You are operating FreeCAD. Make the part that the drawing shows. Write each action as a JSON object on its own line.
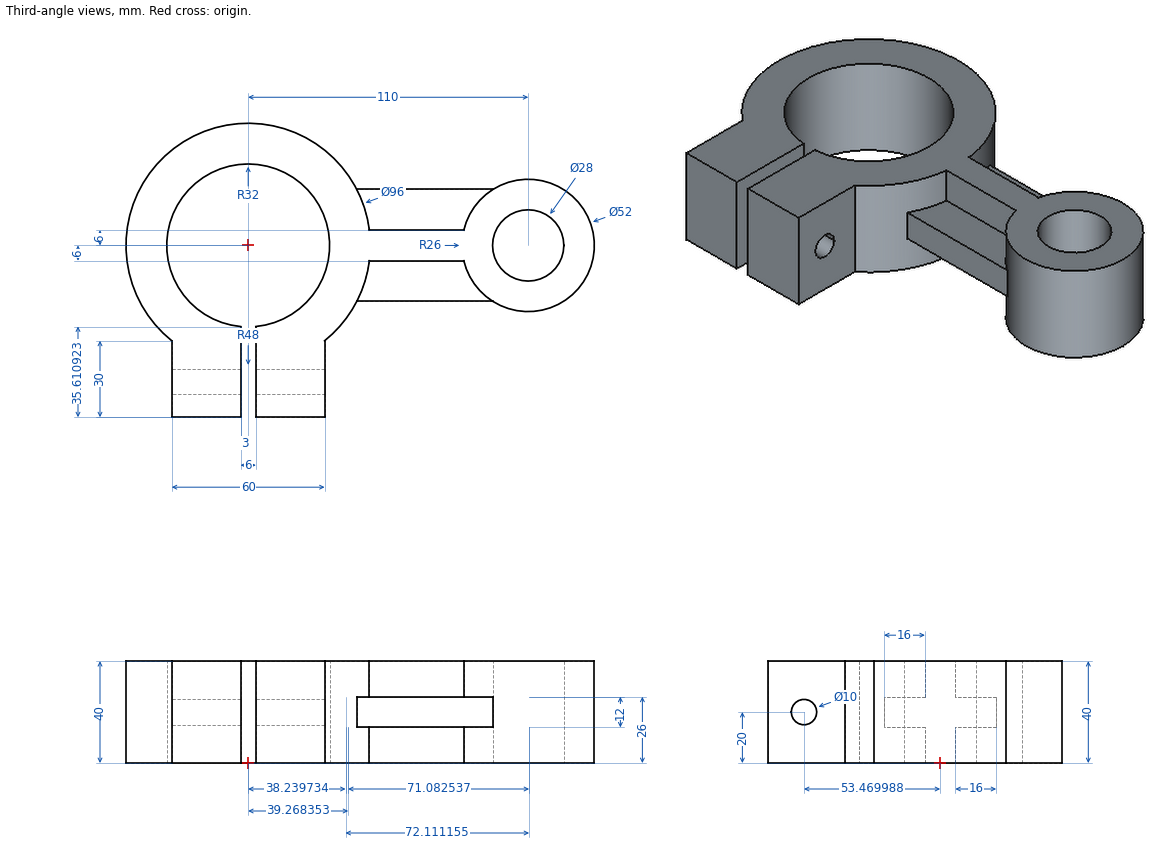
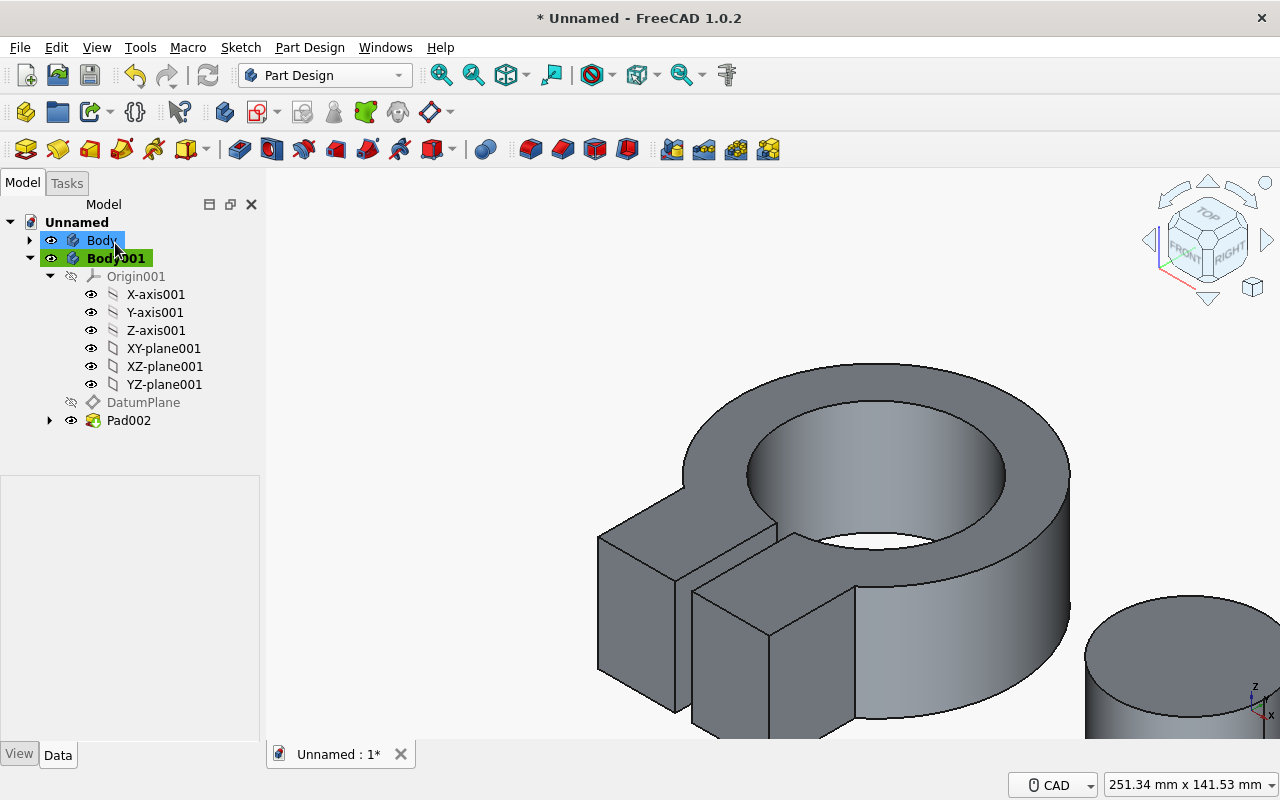
{"action": "left_click", "coordinate": [442, 76]}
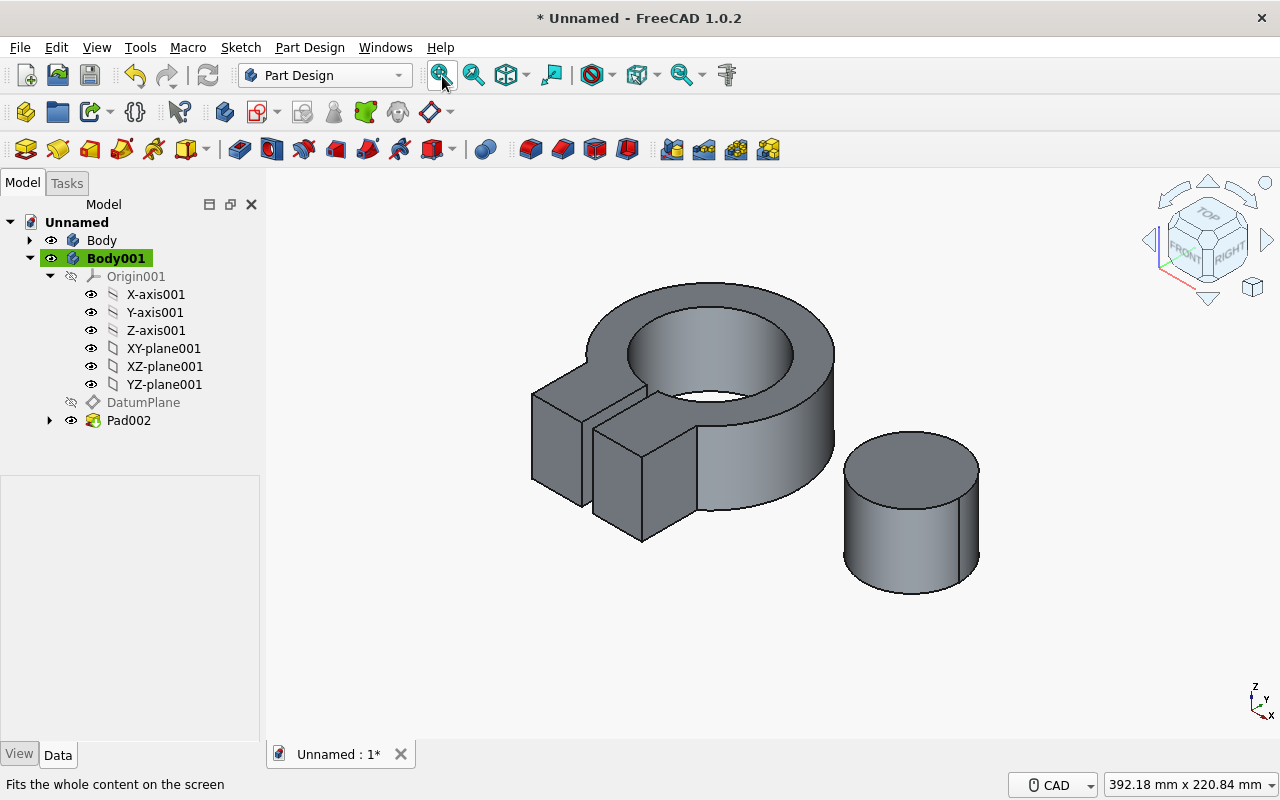
{"action": "double_click", "coordinate": [96, 240]}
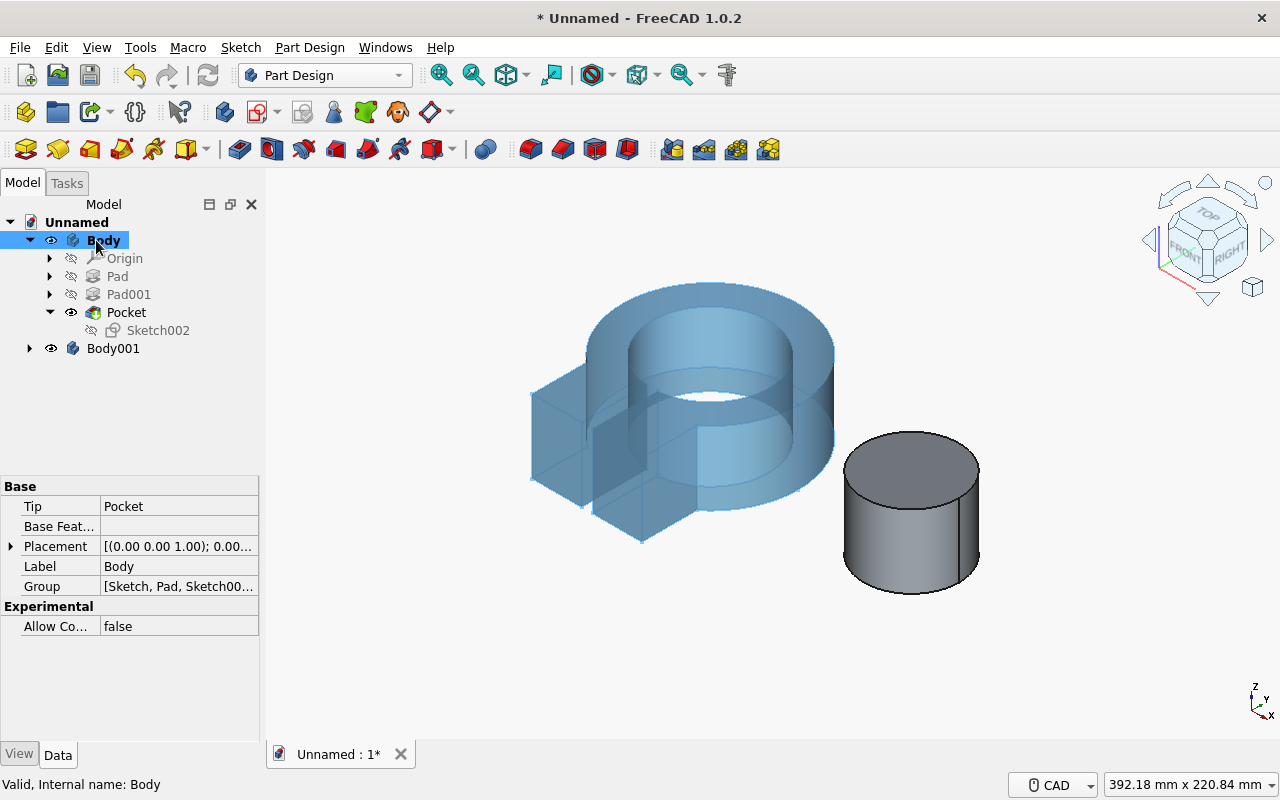
{"action": "left_click", "coordinate": [96, 240]}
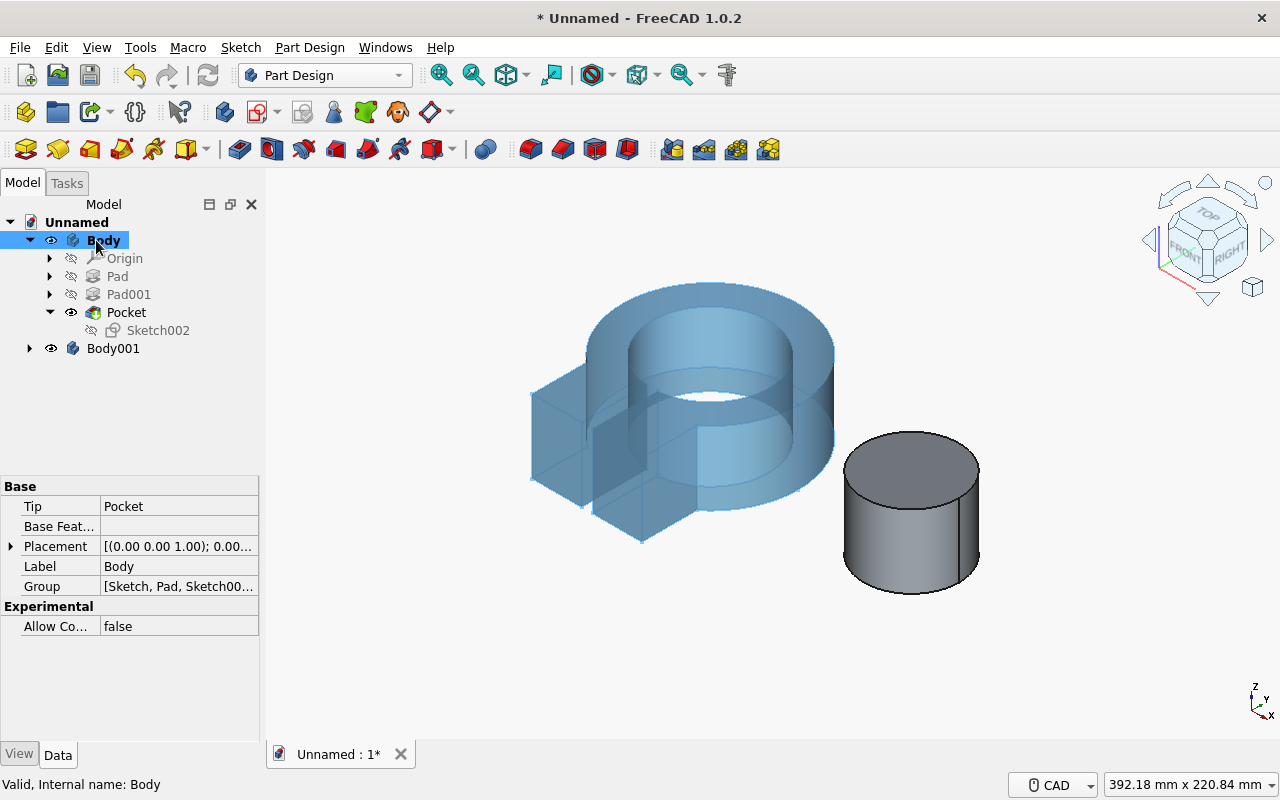
{"action": "left_click", "coordinate": [146, 626]}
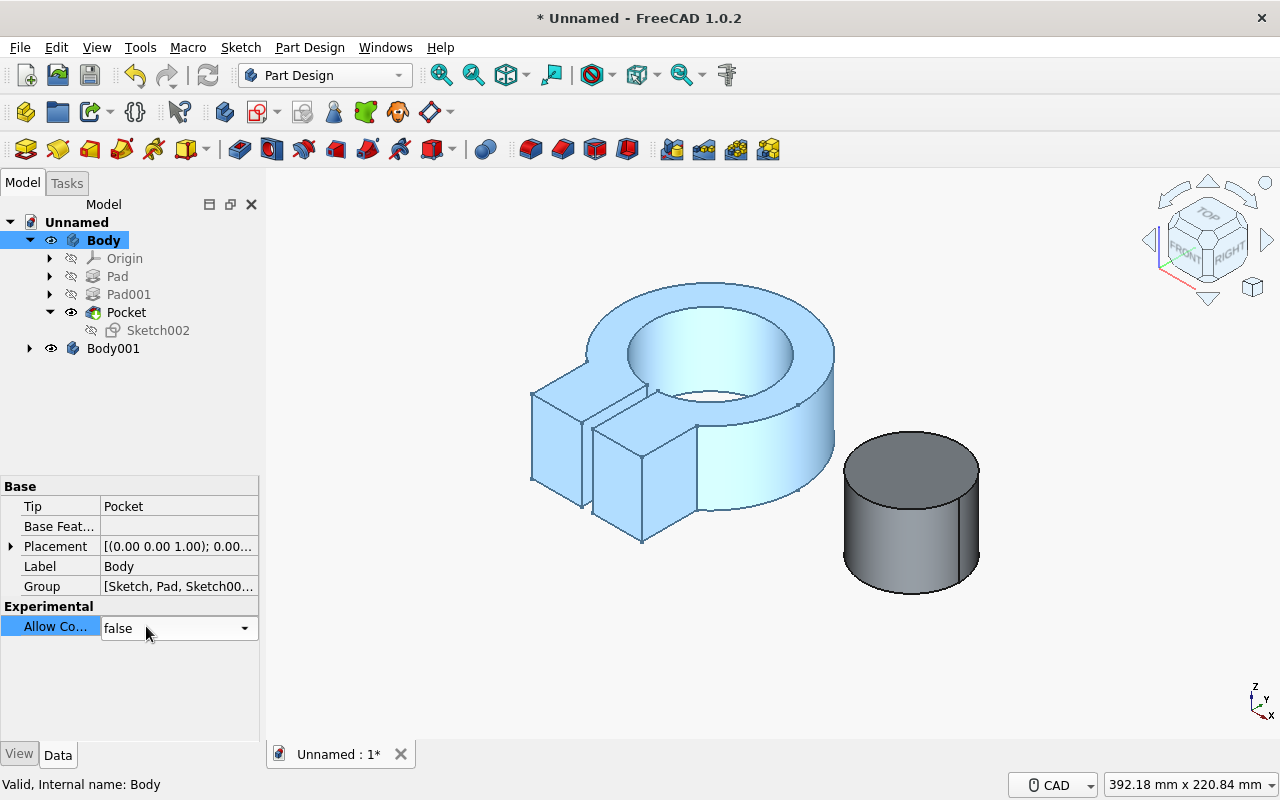
{"action": "left_click", "coordinate": [146, 626]}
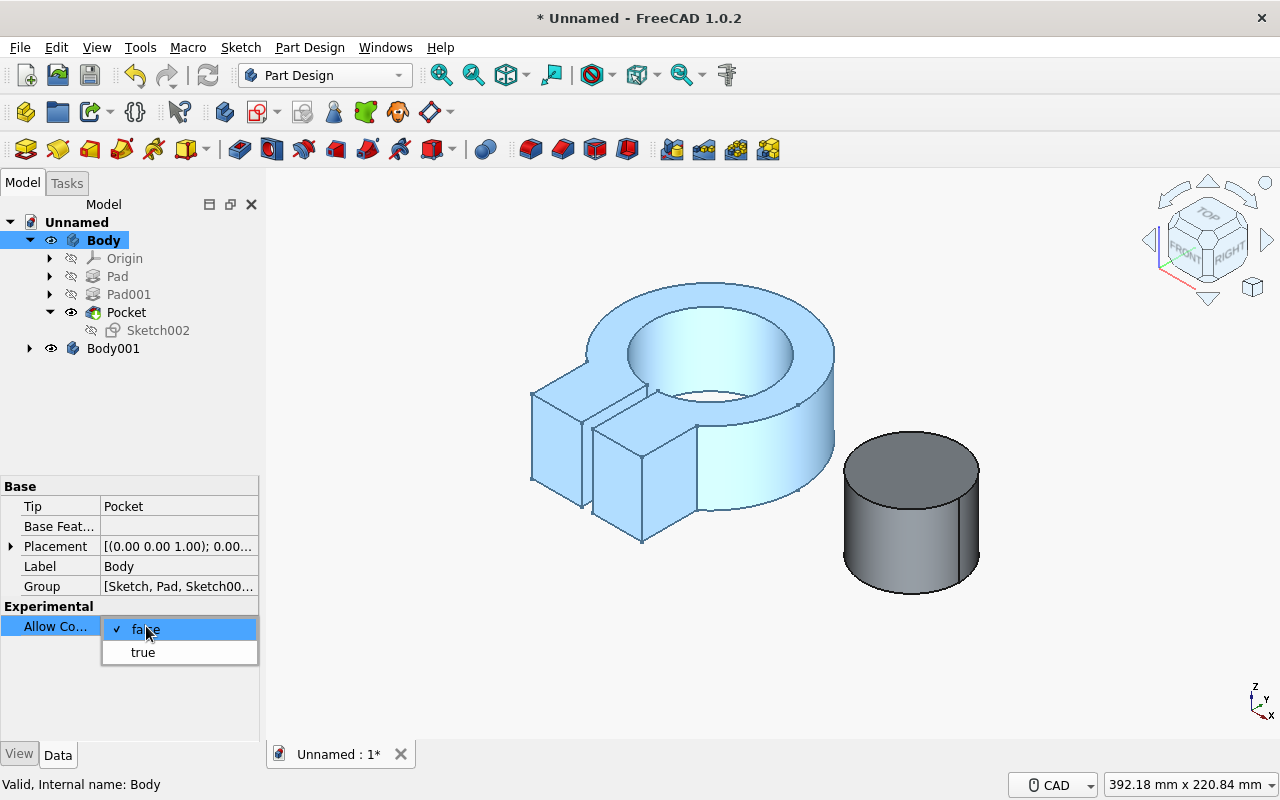
{"action": "left_click", "coordinate": [179, 652]}
{"action": "key", "text": "Return"}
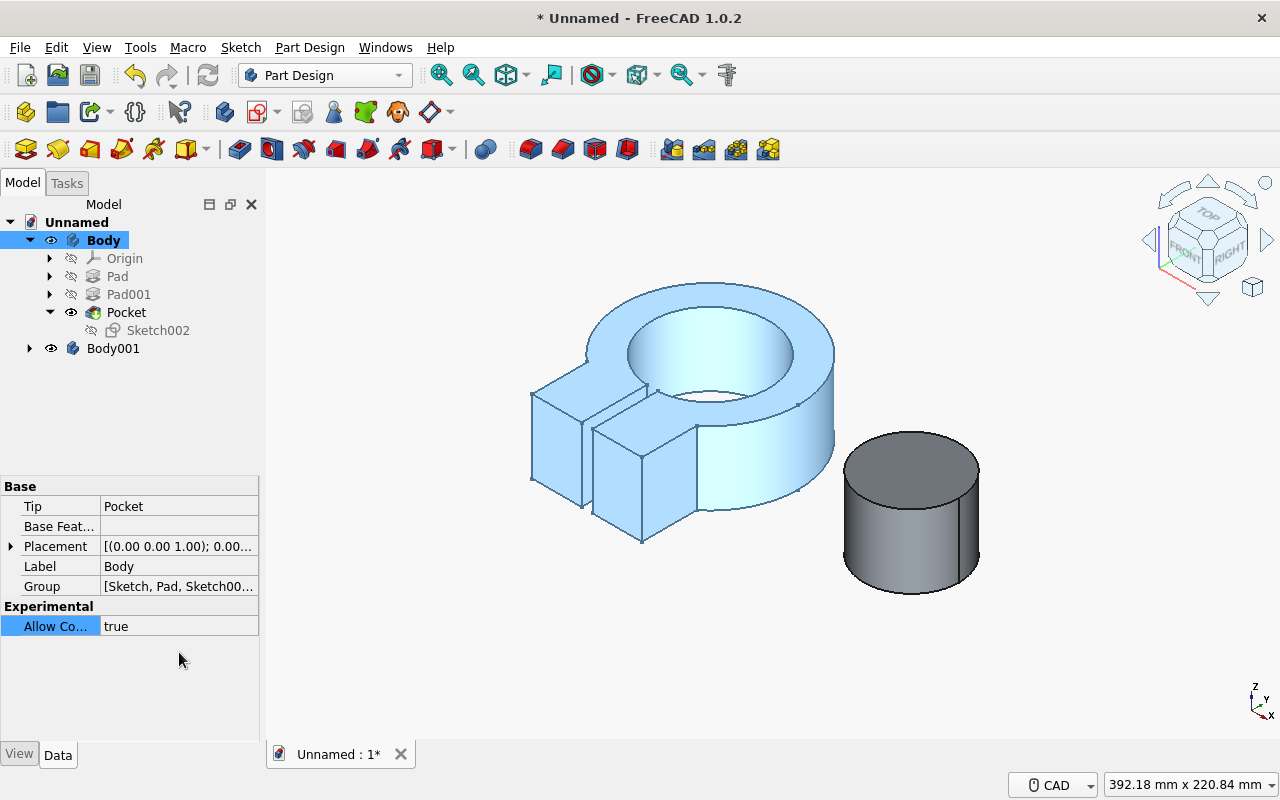
{"action": "left_click", "coordinate": [96, 348]}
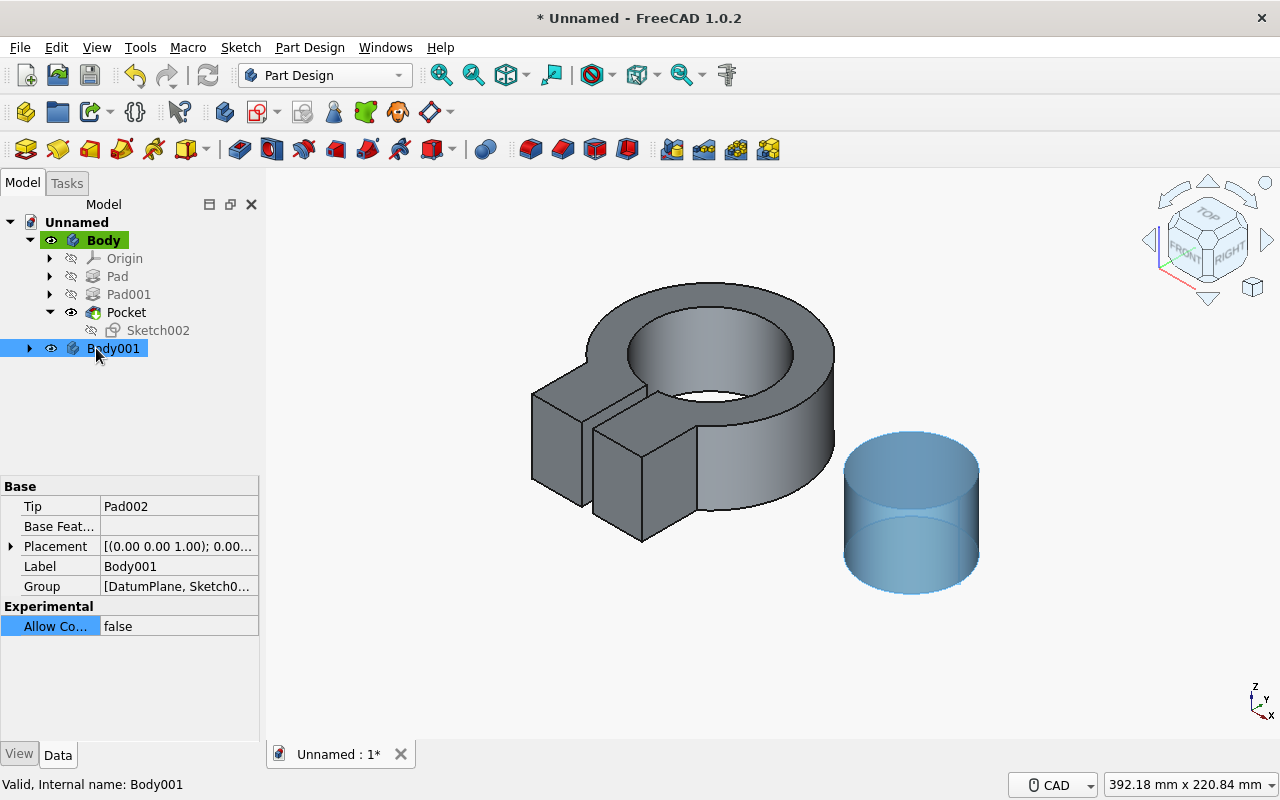
{"action": "left_click", "coordinate": [486, 150]}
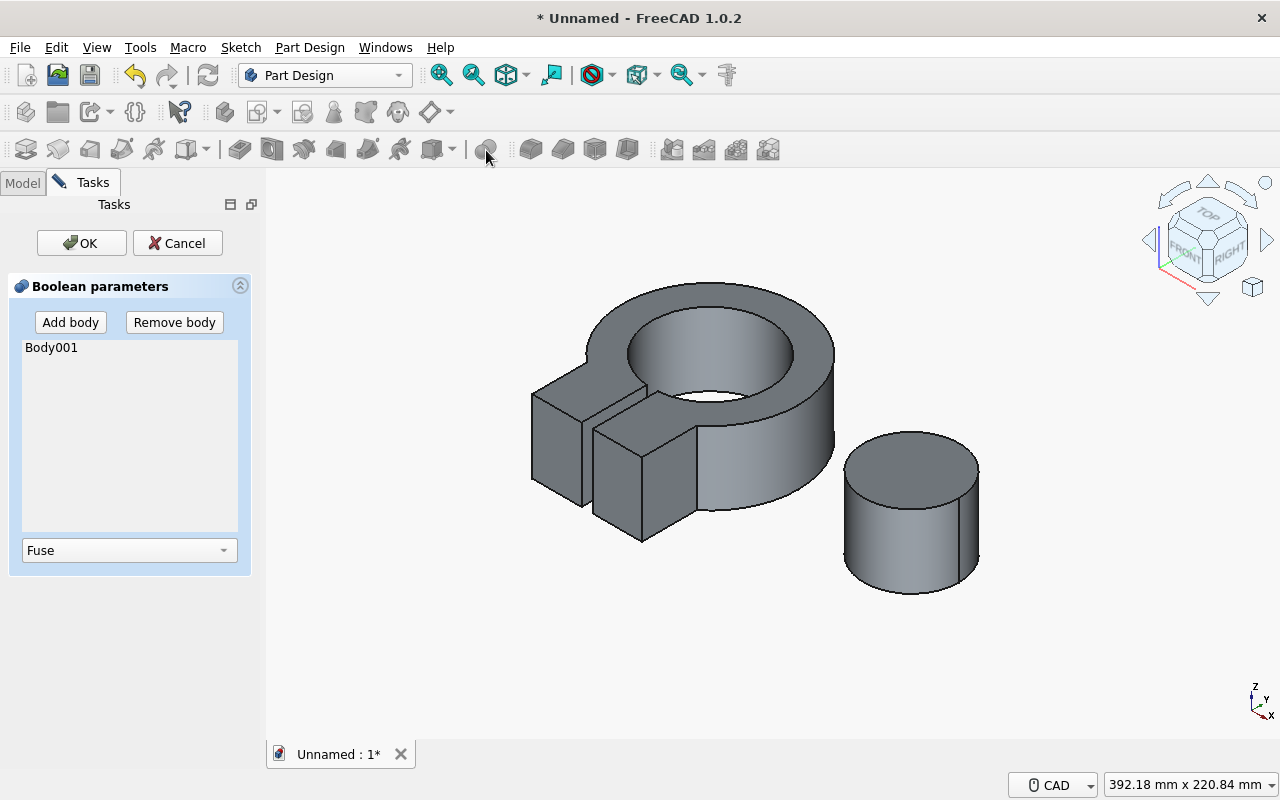
{"action": "left_click", "coordinate": [82, 243]}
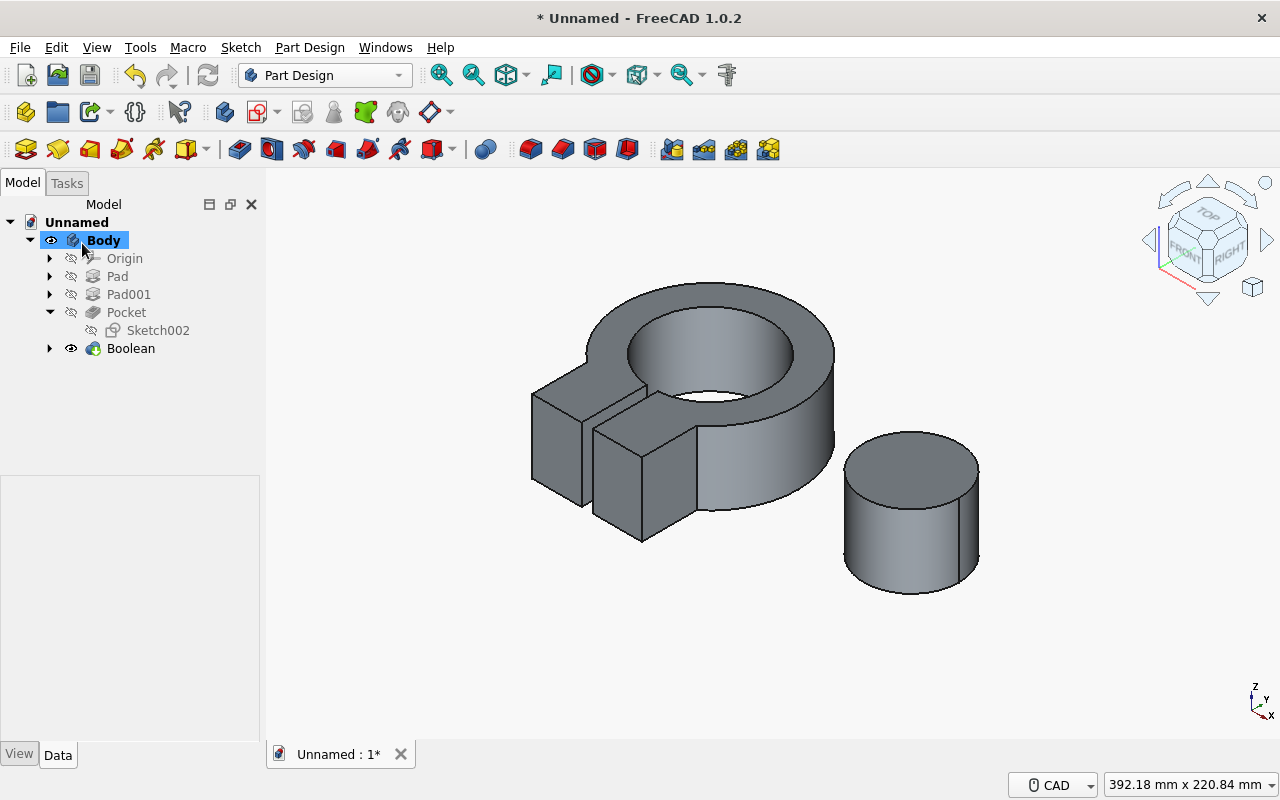
{"action": "left_click", "coordinate": [258, 112]}